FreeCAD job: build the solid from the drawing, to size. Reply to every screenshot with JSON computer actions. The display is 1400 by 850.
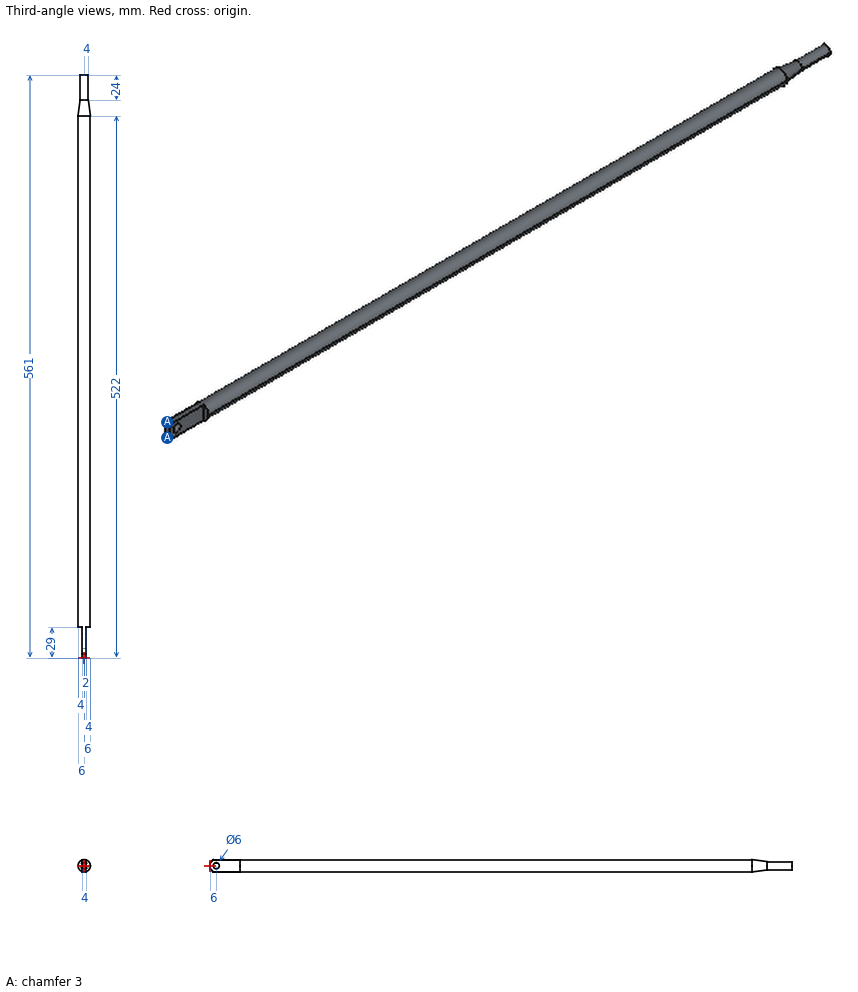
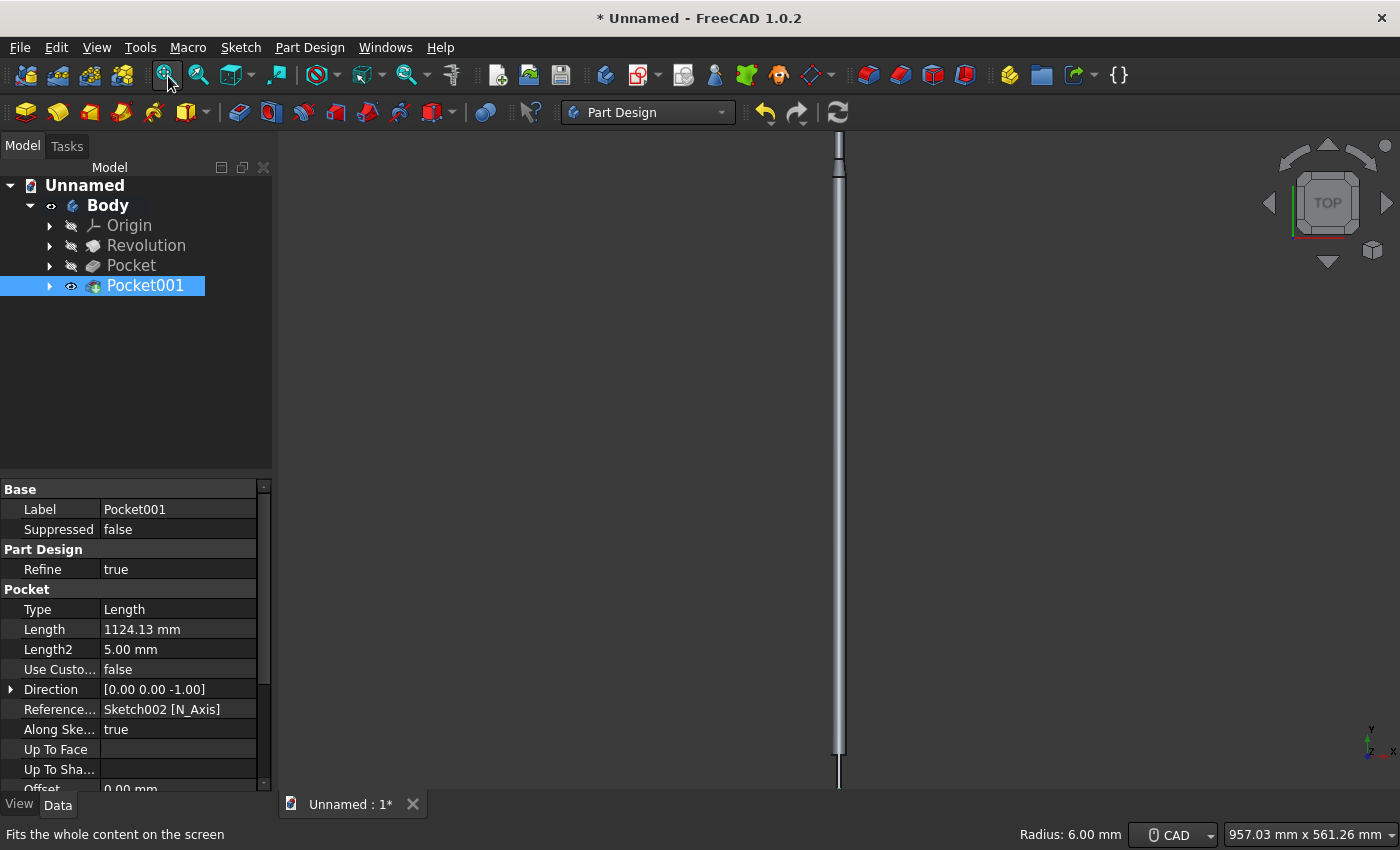
{"action": "key", "text": "1"}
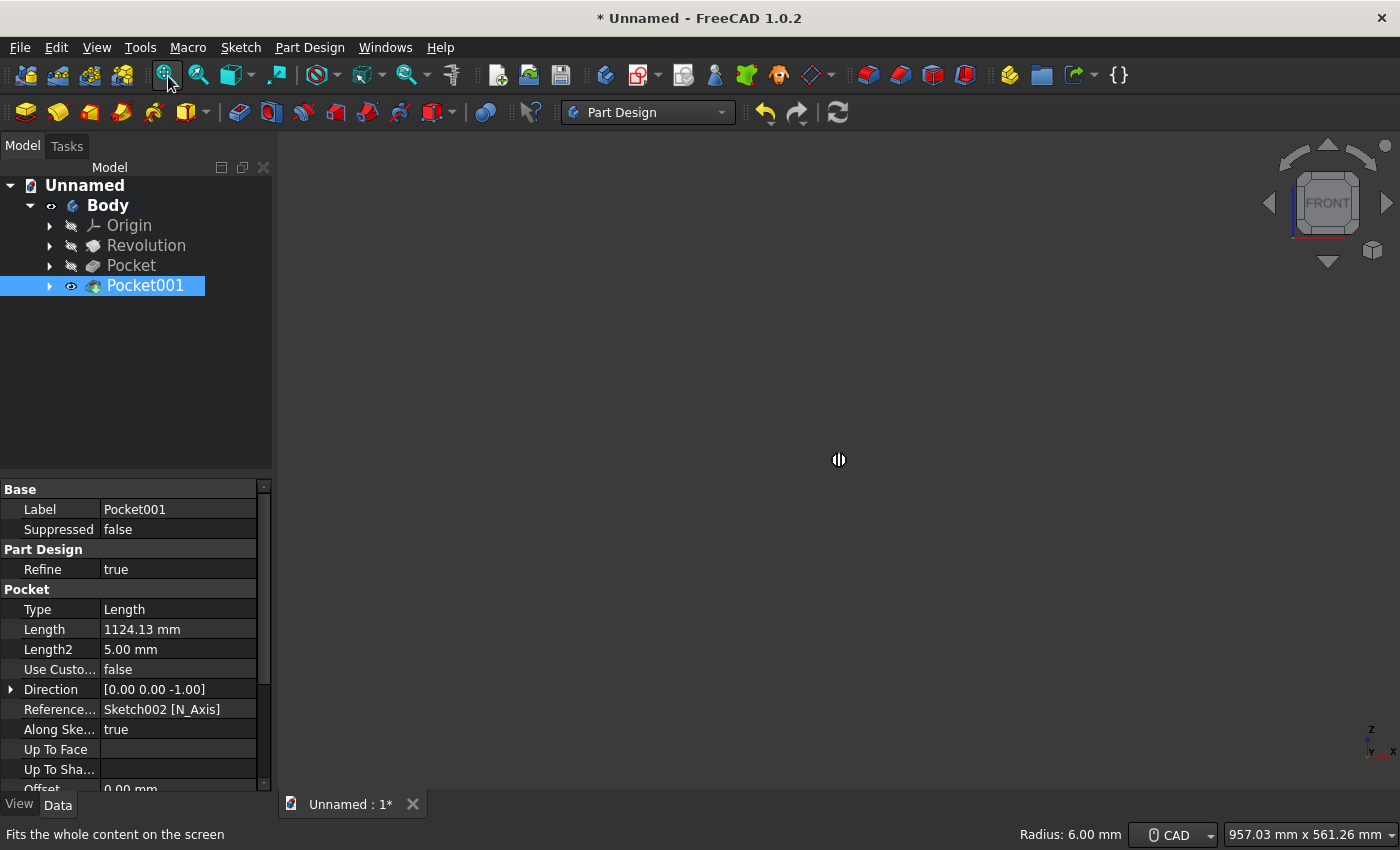
{"action": "left_click", "coordinate": [168, 76]}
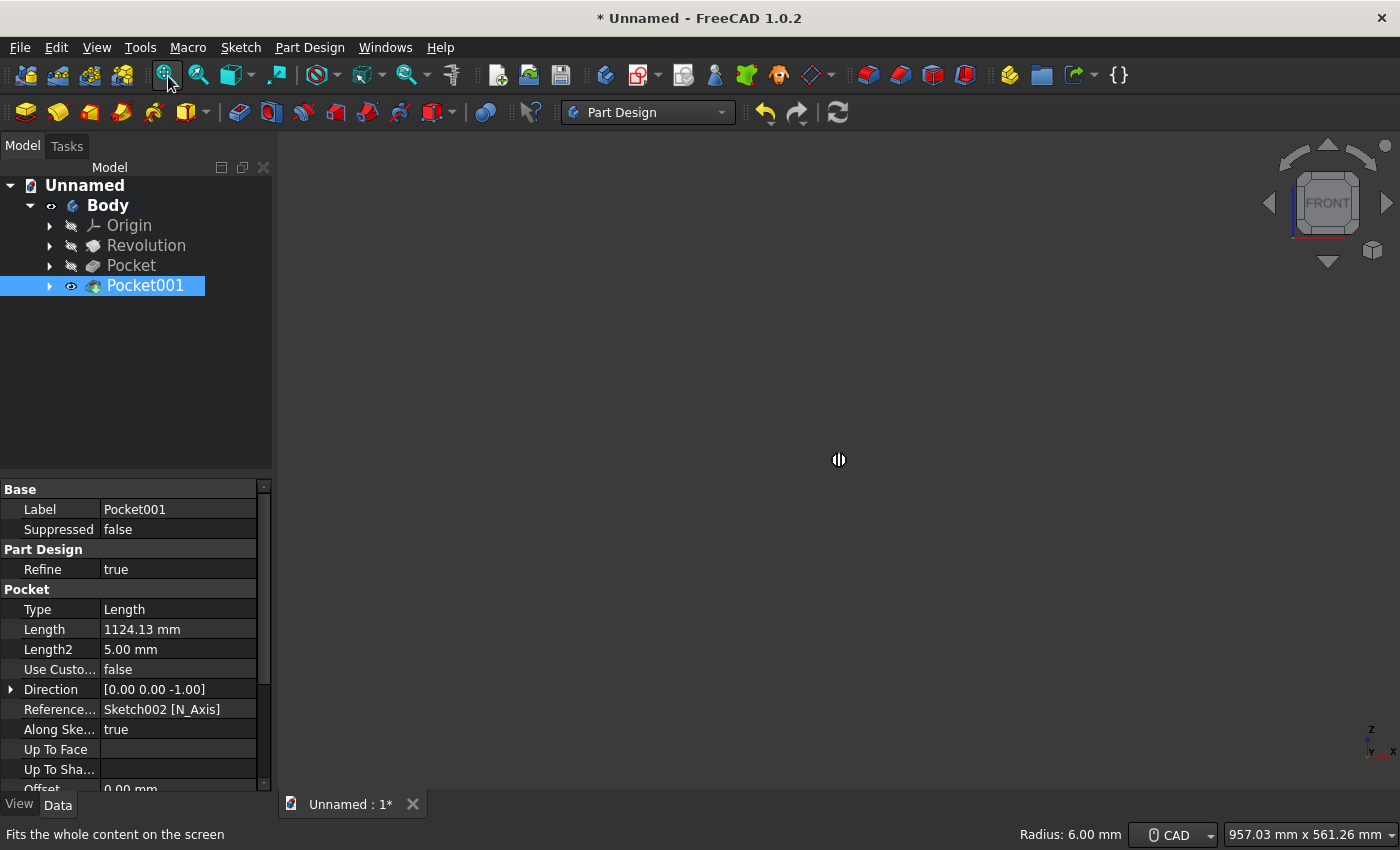
{"action": "scroll", "coordinate": [839, 466], "scroll_direction": "up", "scroll_amount": 11}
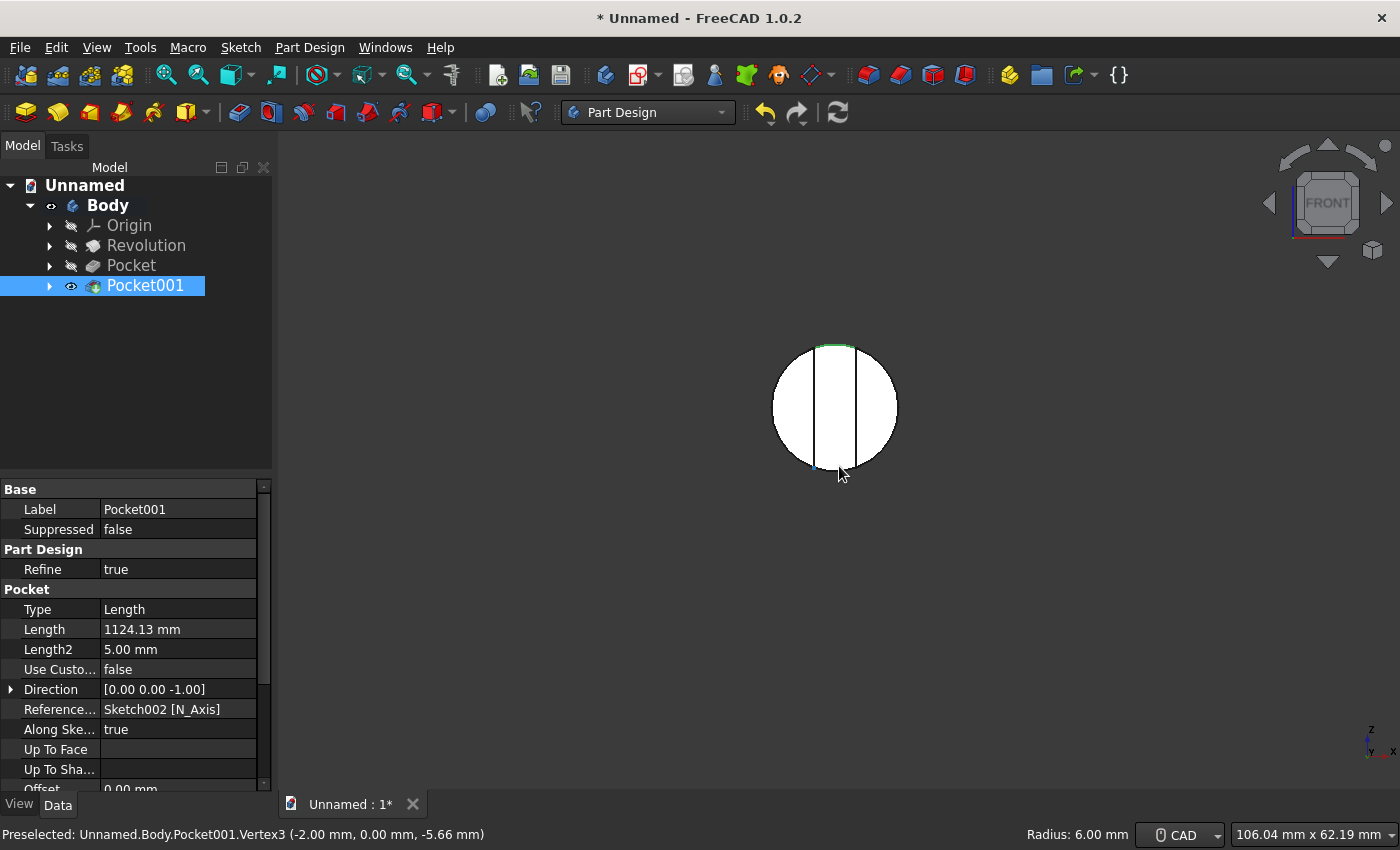
{"action": "left_click", "coordinate": [835, 470], "text": "ctrl"}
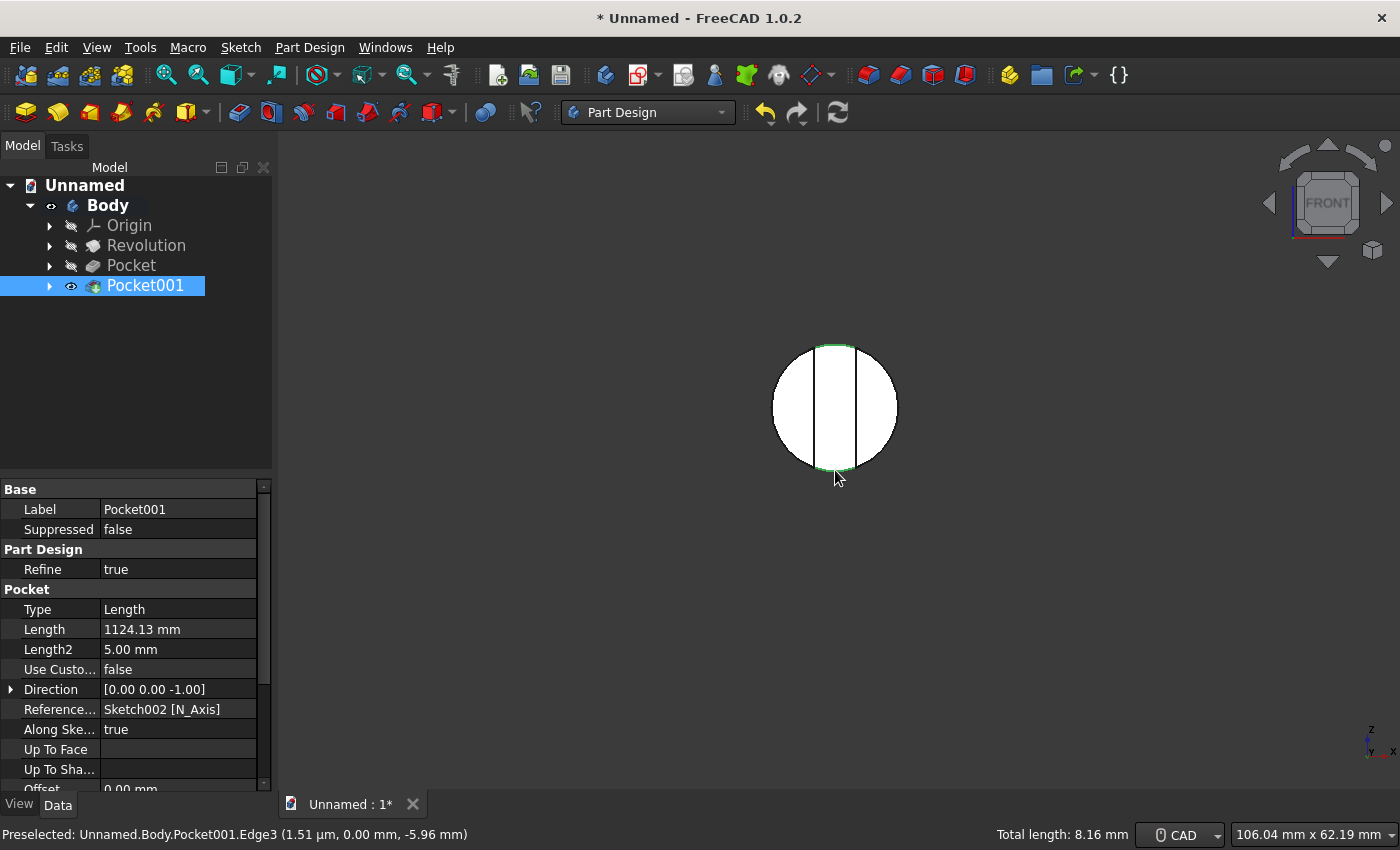
{"action": "left_click", "coordinate": [902, 76]}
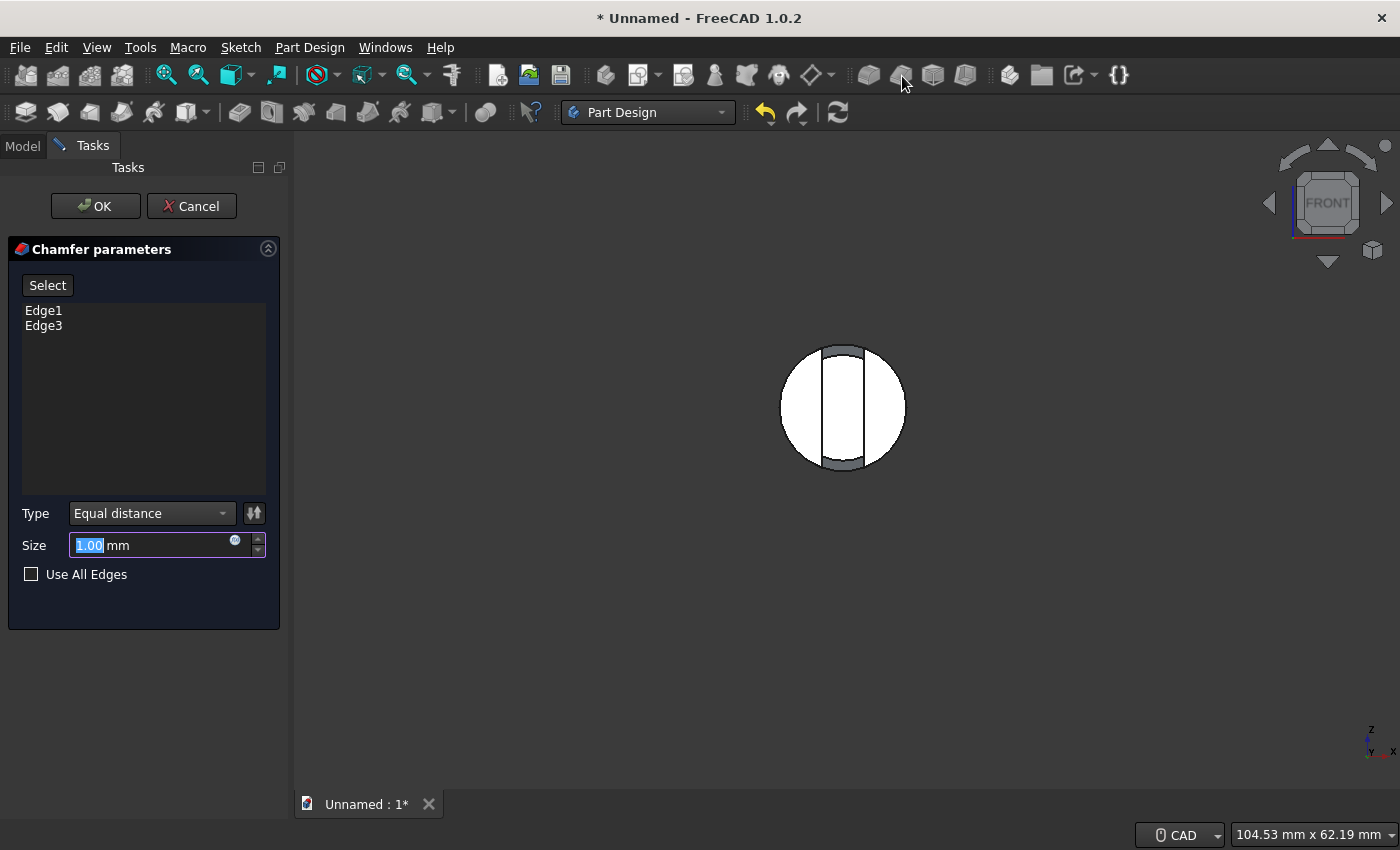
{"action": "type", "text": "3"}
{"action": "key", "text": "Tab"}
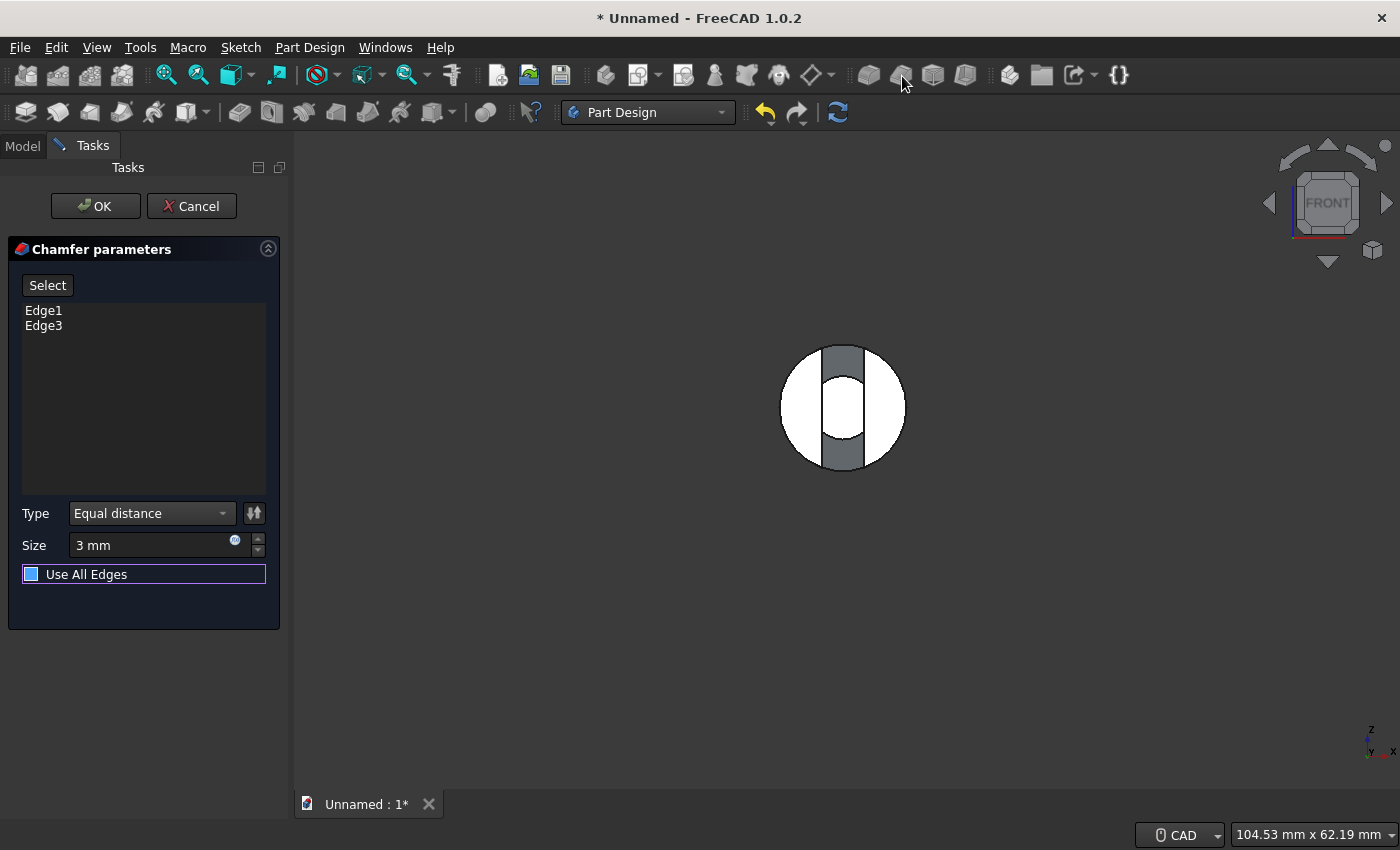
{"action": "left_click", "coordinate": [96, 206]}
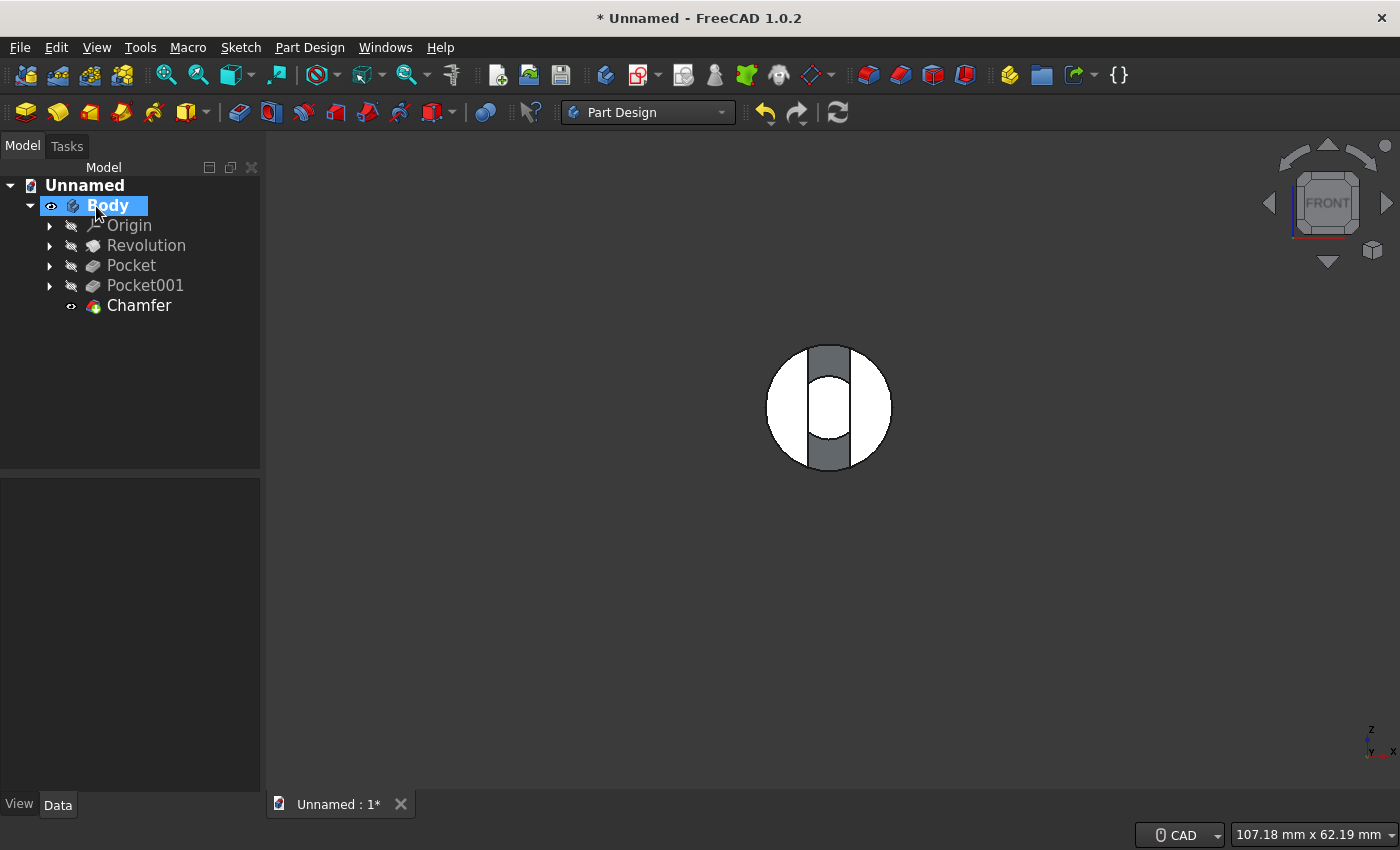
{"action": "left_click", "coordinate": [168, 76]}